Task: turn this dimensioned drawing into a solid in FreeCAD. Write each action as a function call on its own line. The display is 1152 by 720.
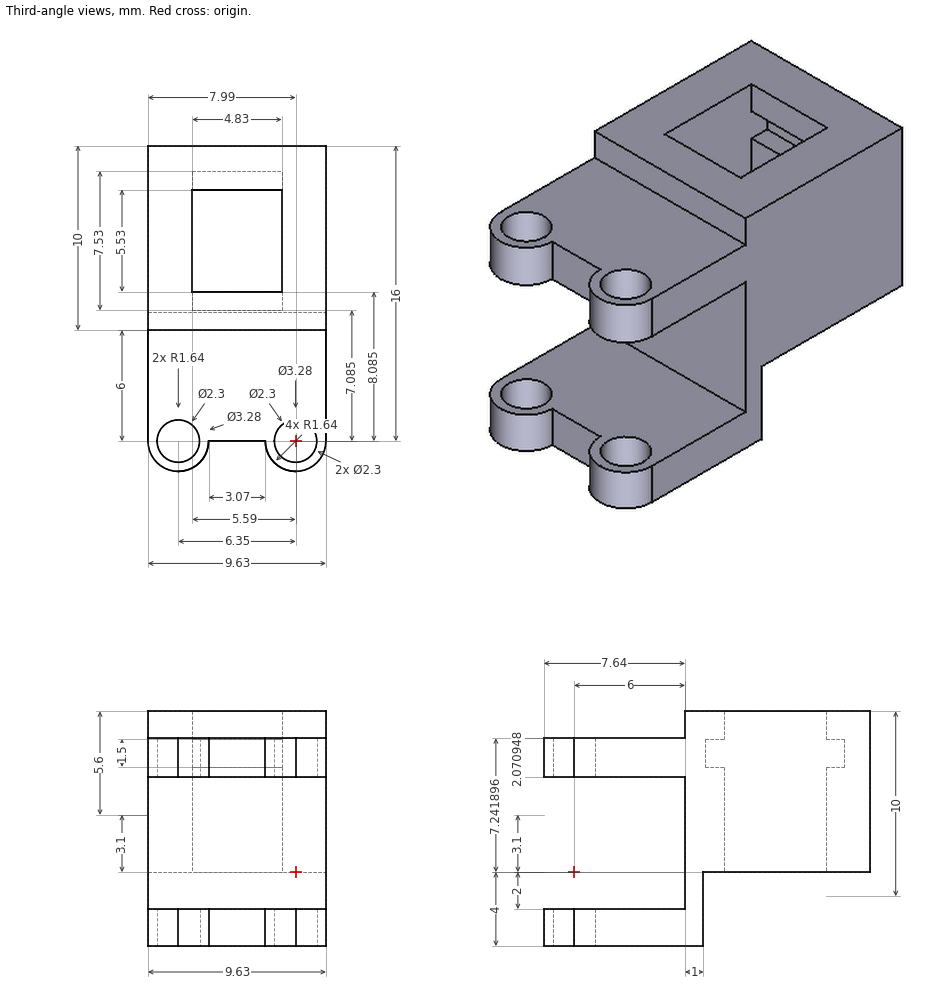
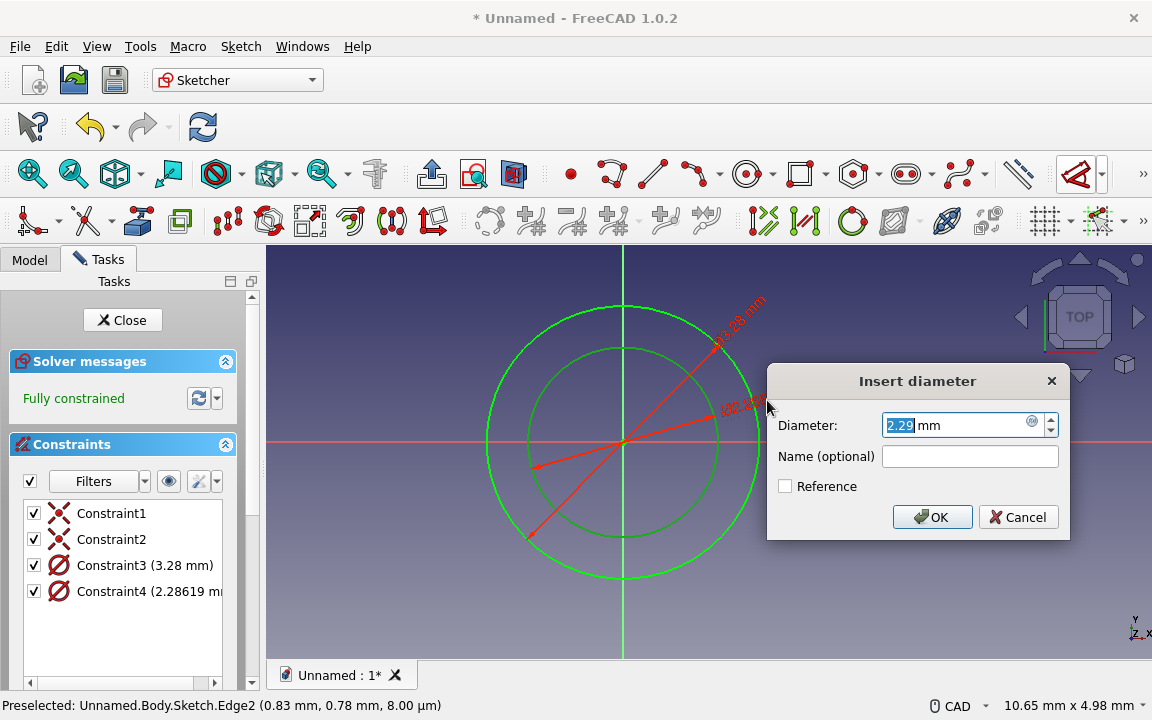
text(2.3)
key(Return)
key(Escape)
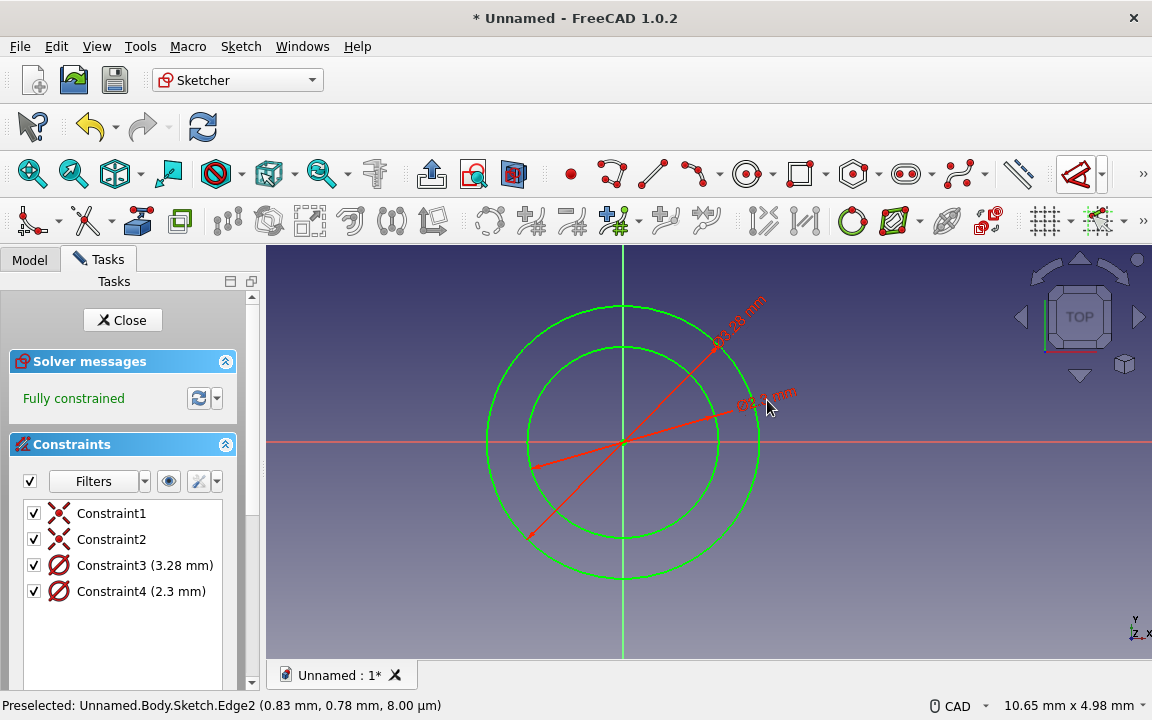
click(123, 320)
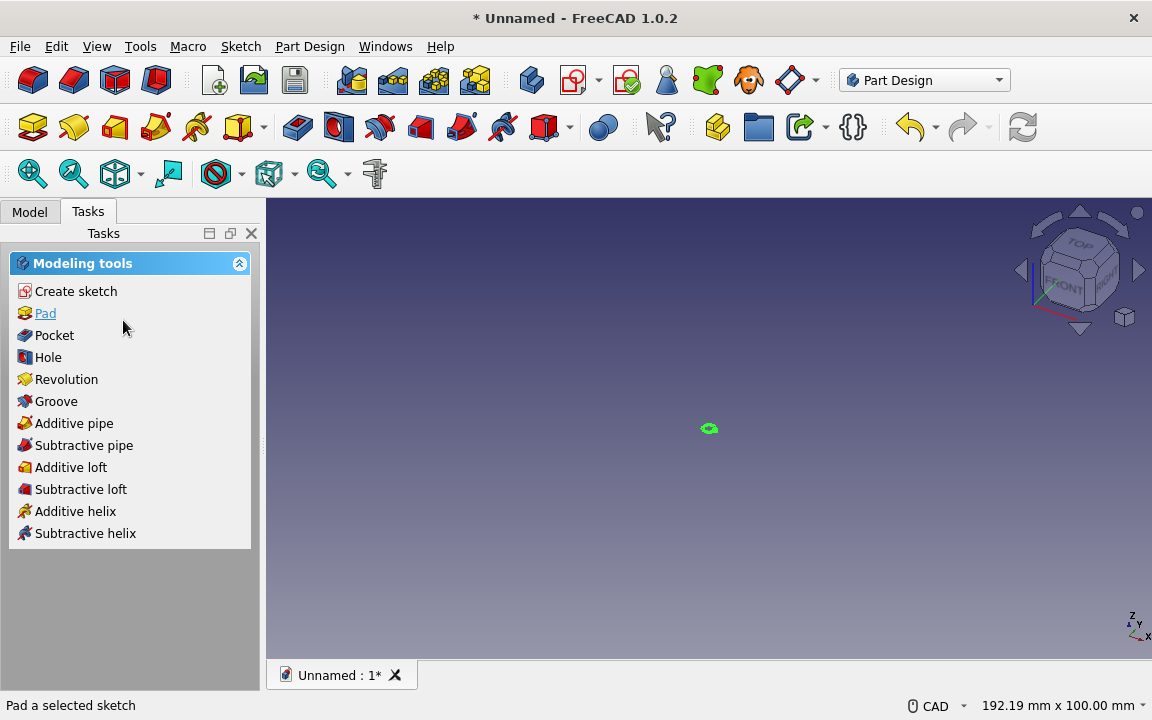
click(33, 128)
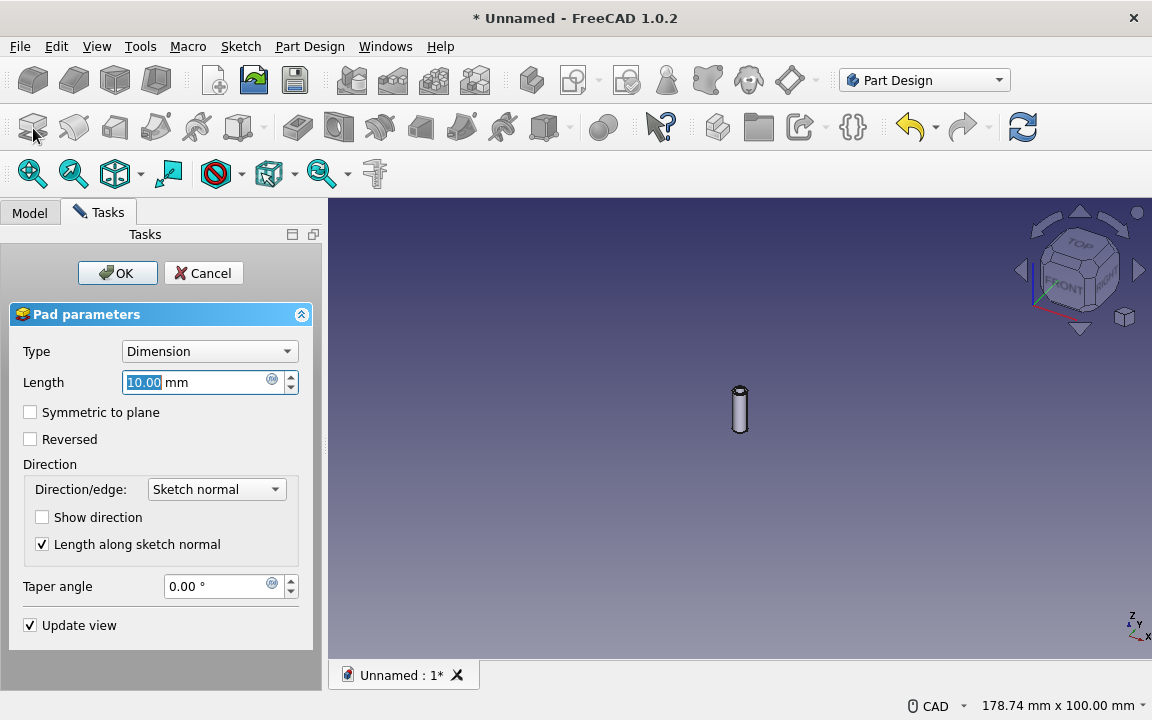
text(3.1)
key(Tab)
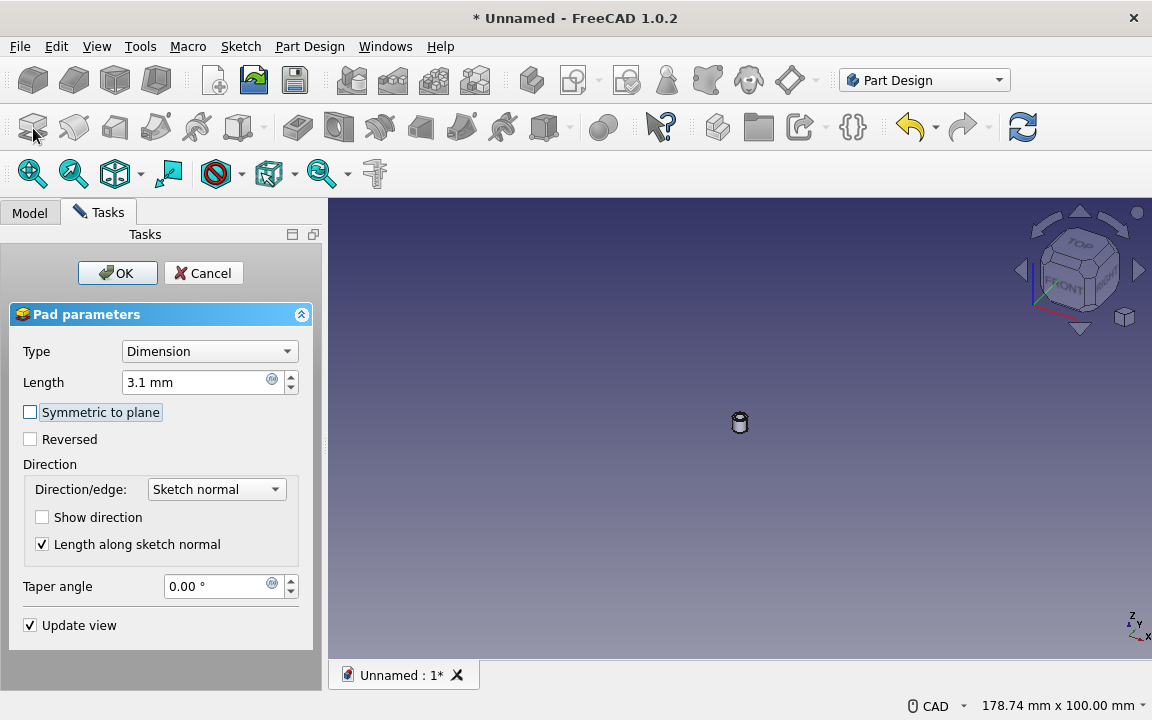
click(118, 273)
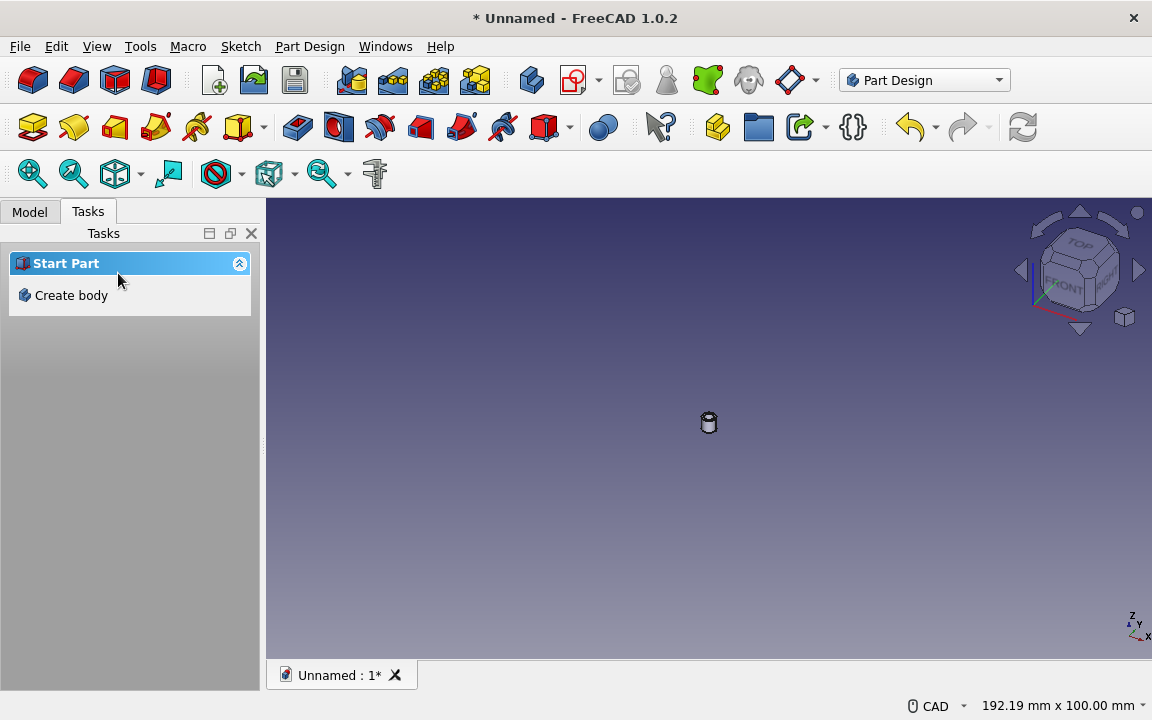
click(33, 174)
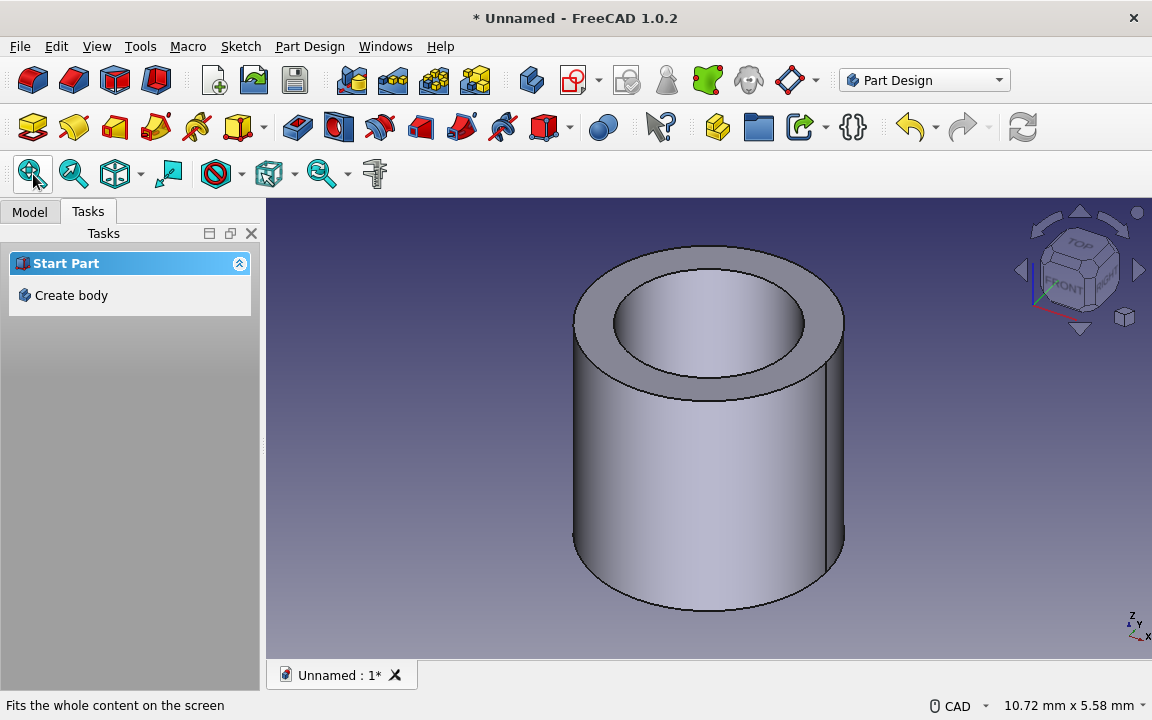
click(532, 80)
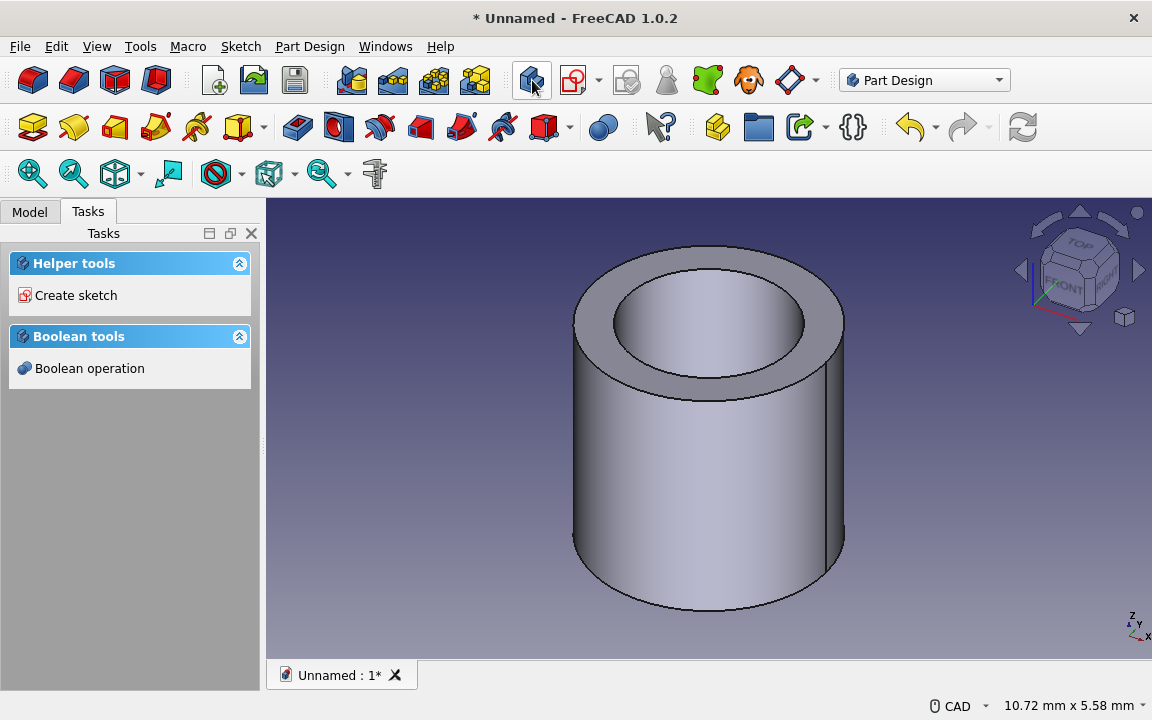
click(306, 619)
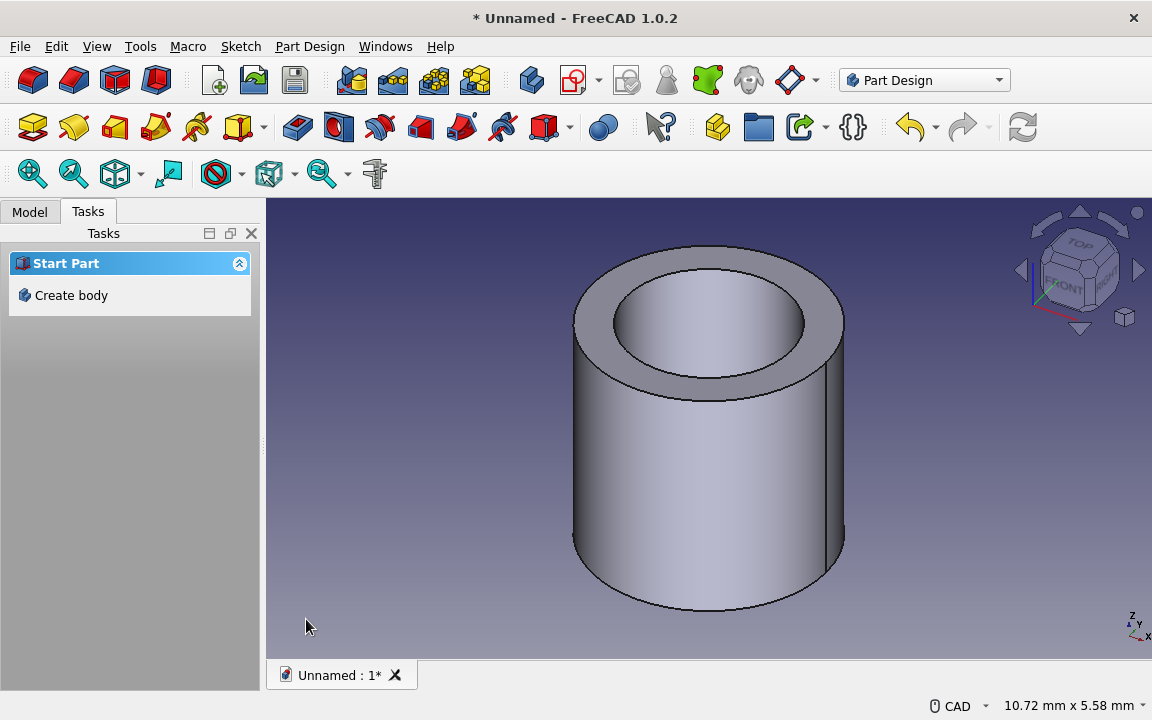
click(572, 80)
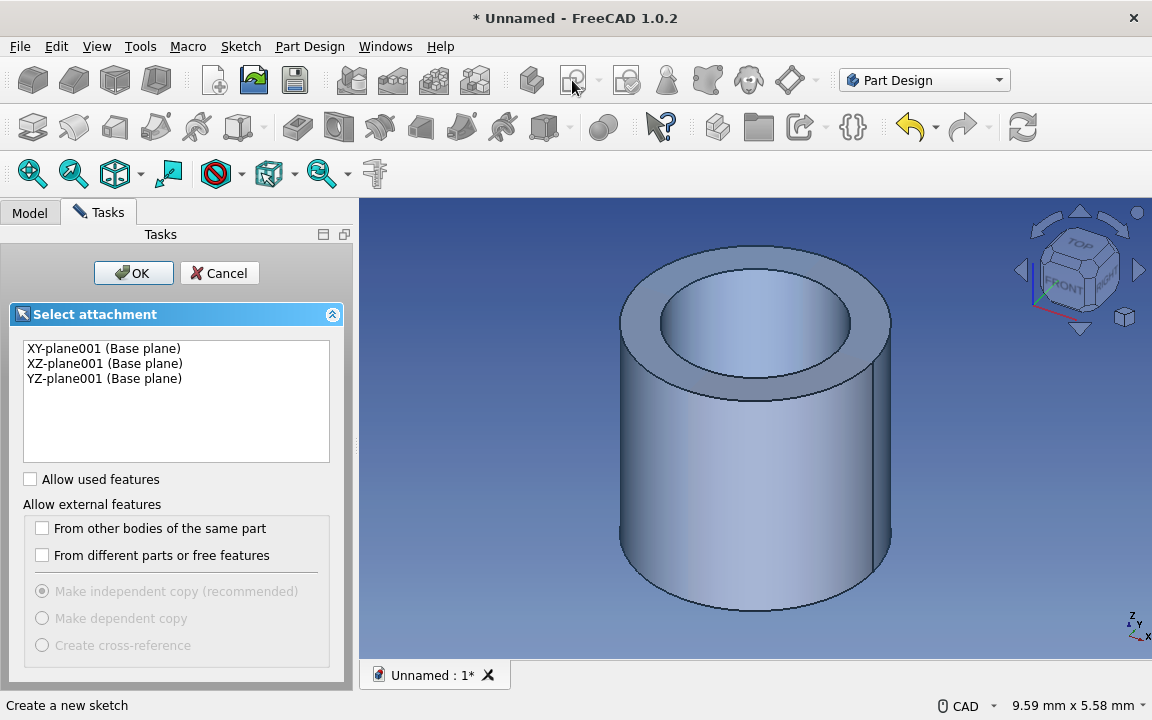
click(84, 348)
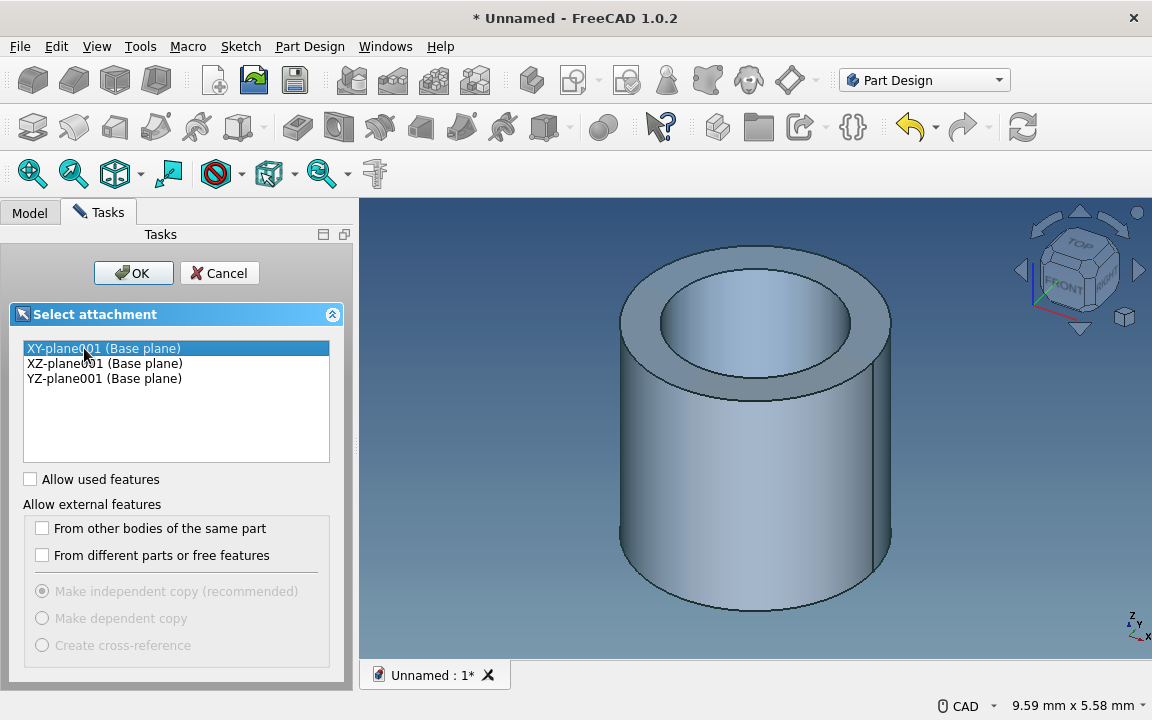
click(134, 273)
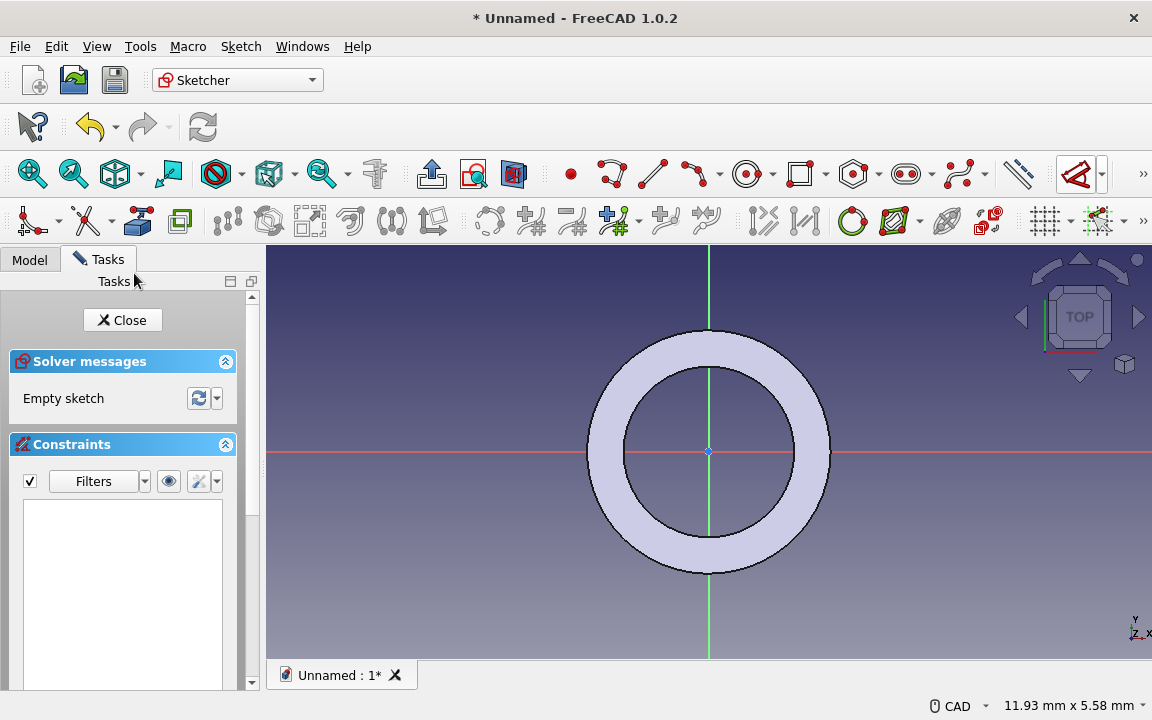
scroll(987, 452, down, 2)